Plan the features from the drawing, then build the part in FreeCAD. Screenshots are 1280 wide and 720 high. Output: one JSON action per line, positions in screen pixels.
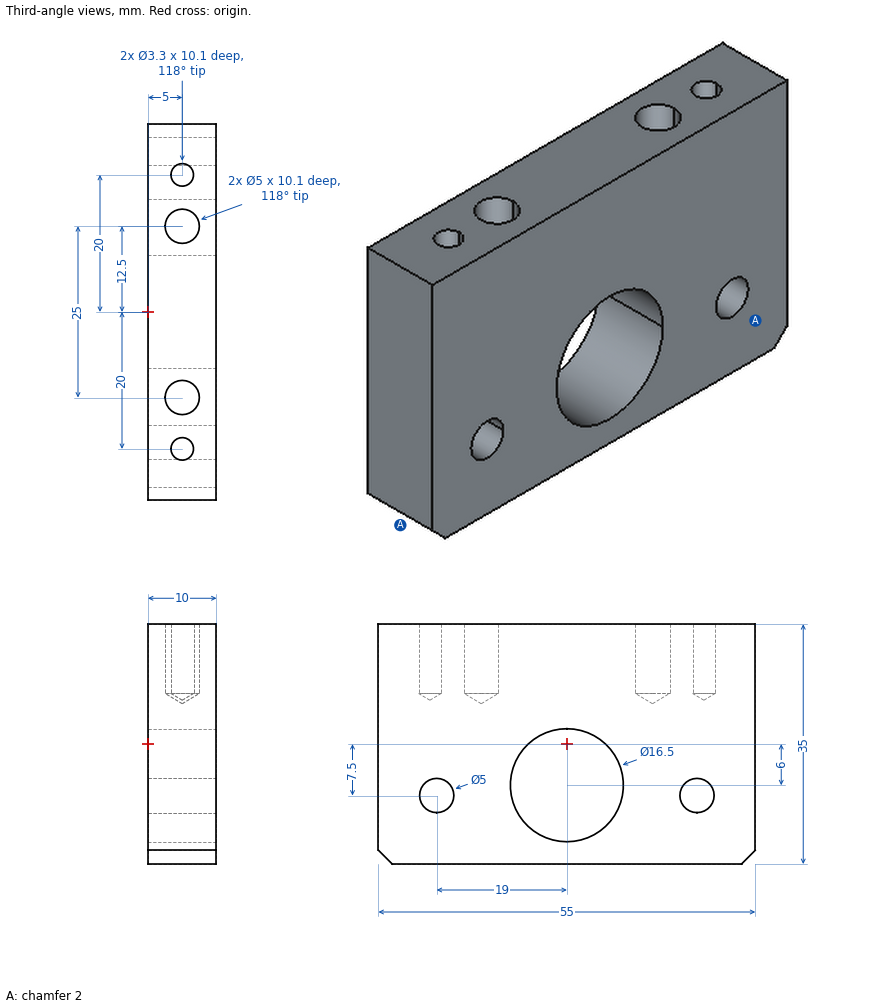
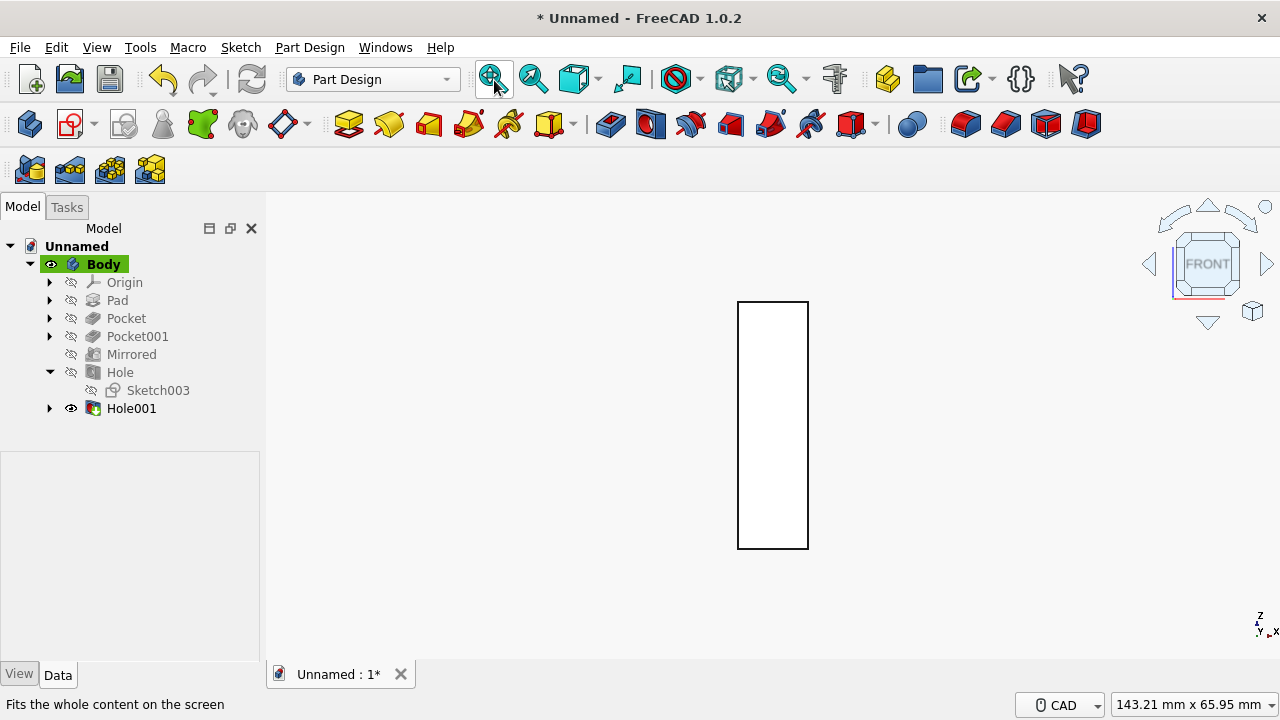
{"action": "left_click", "coordinate": [773, 548]}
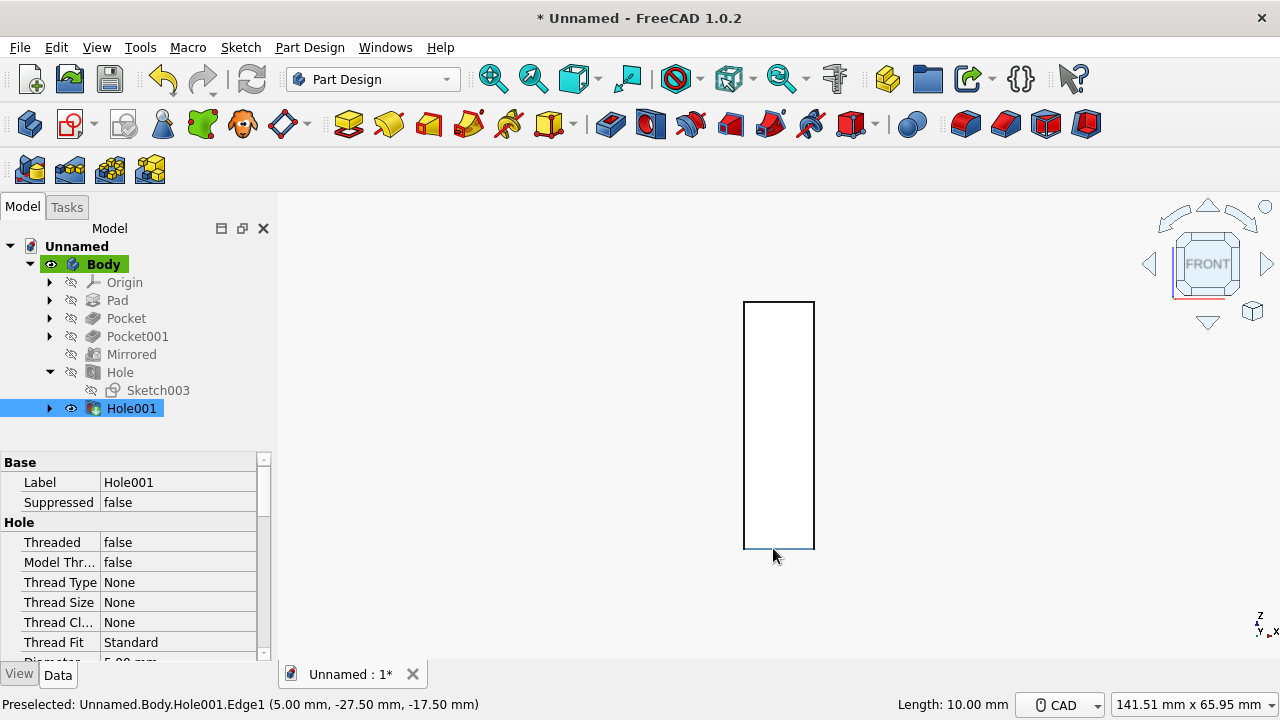
{"action": "key", "text": "3"}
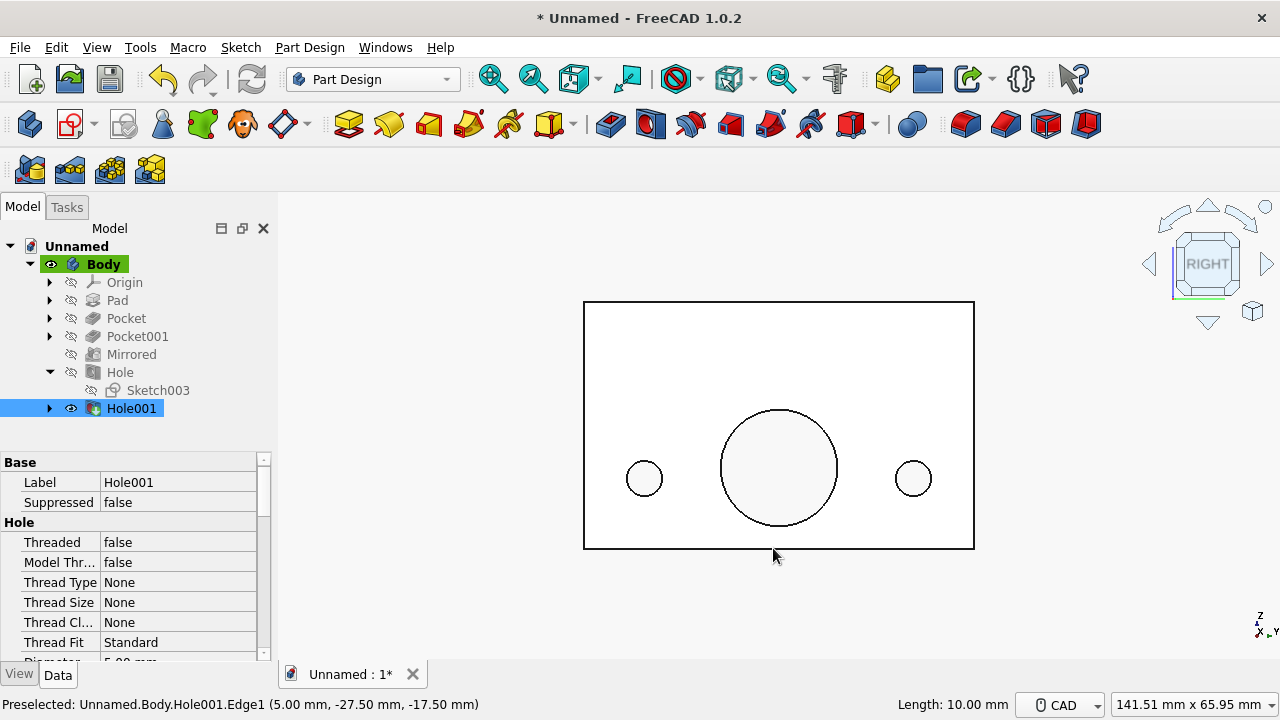
{"action": "key", "text": "5"}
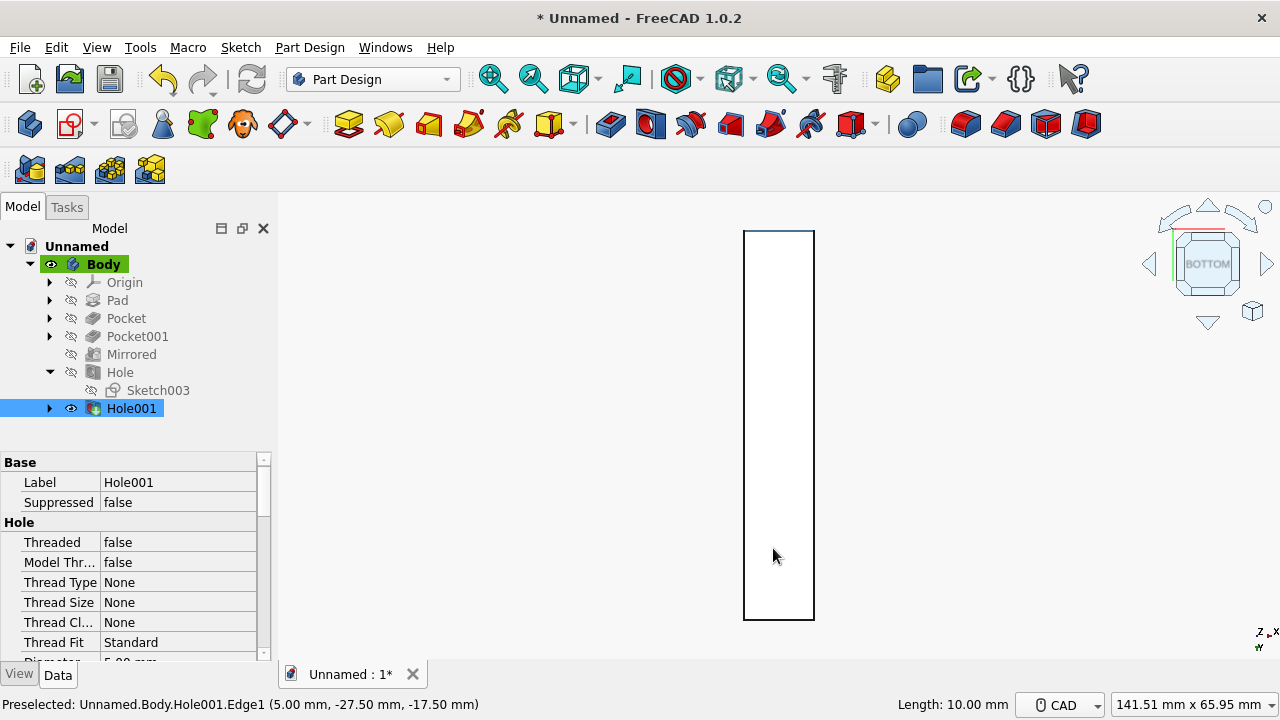
{"action": "left_click", "coordinate": [779, 619], "text": "ctrl"}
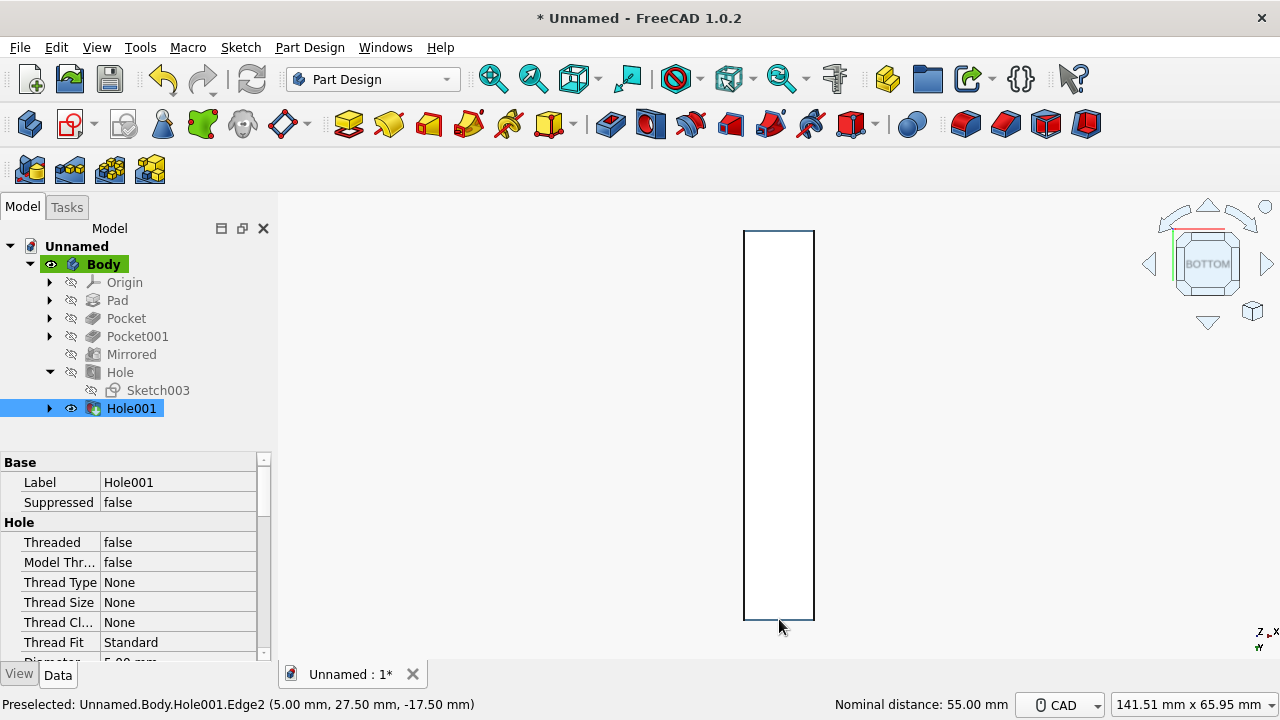
{"action": "left_click", "coordinate": [1006, 124]}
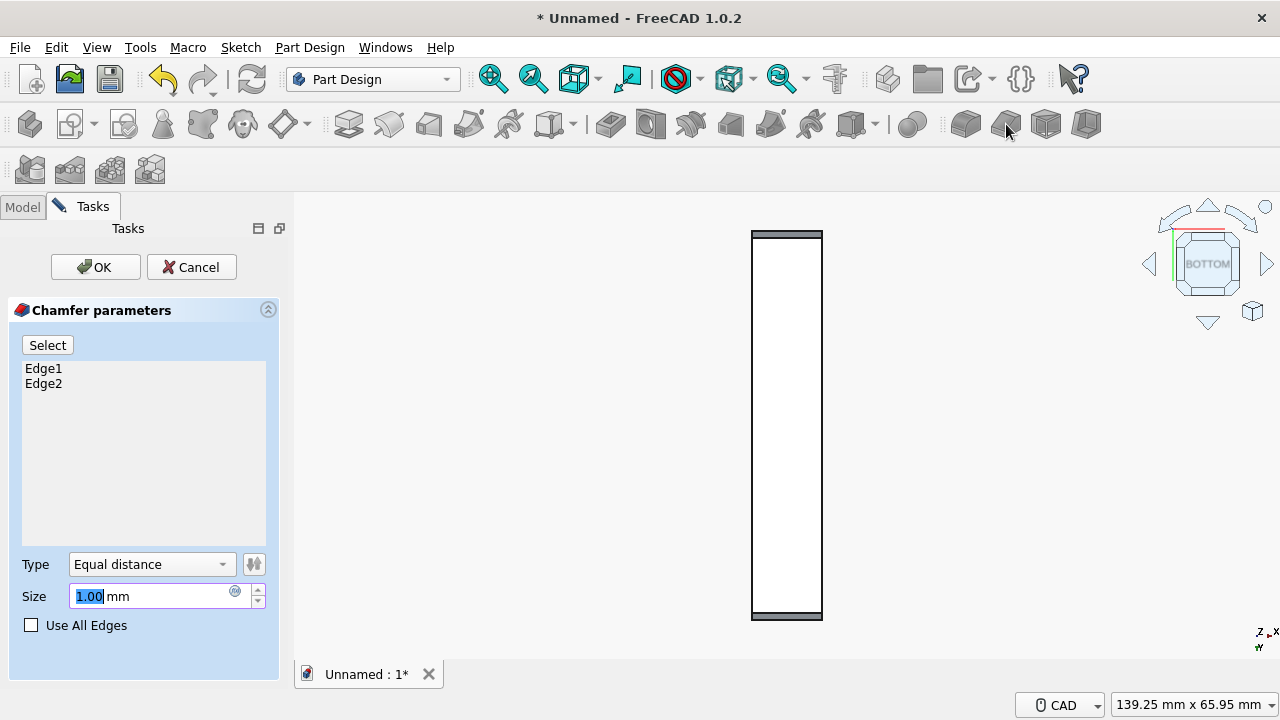
{"action": "type", "text": "2"}
{"action": "key", "text": "Tab"}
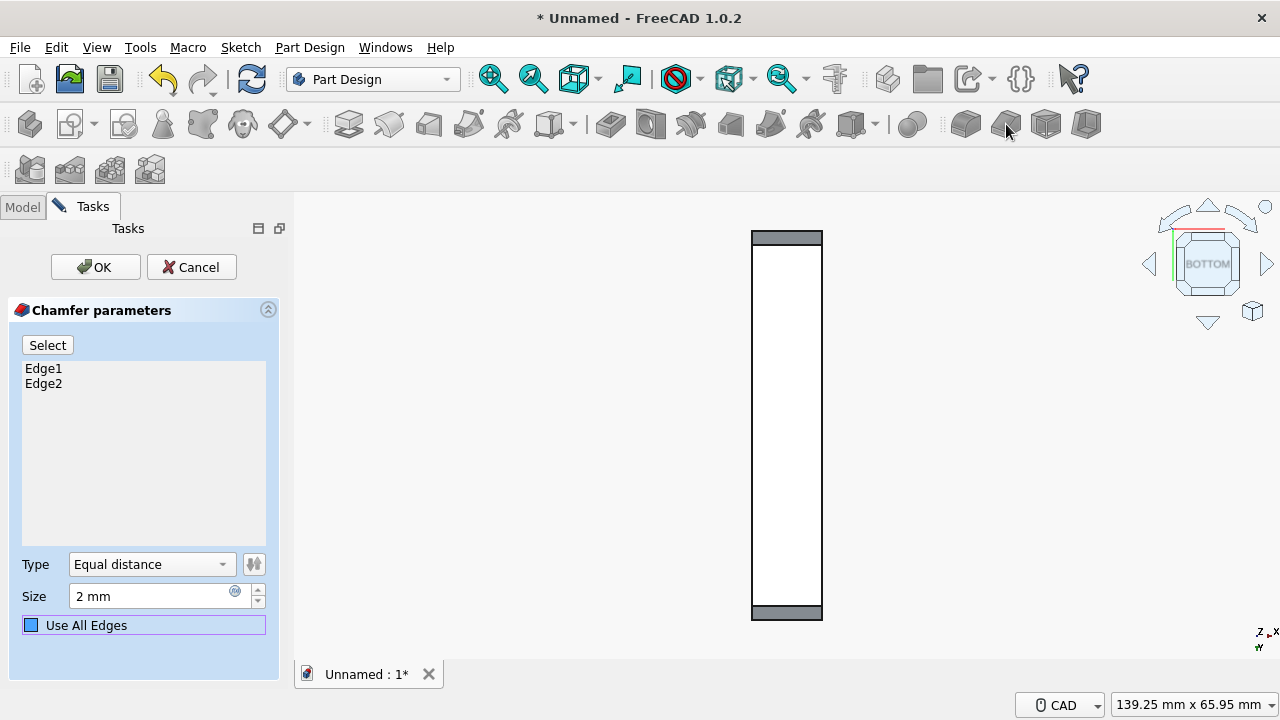
{"action": "left_click", "coordinate": [96, 267]}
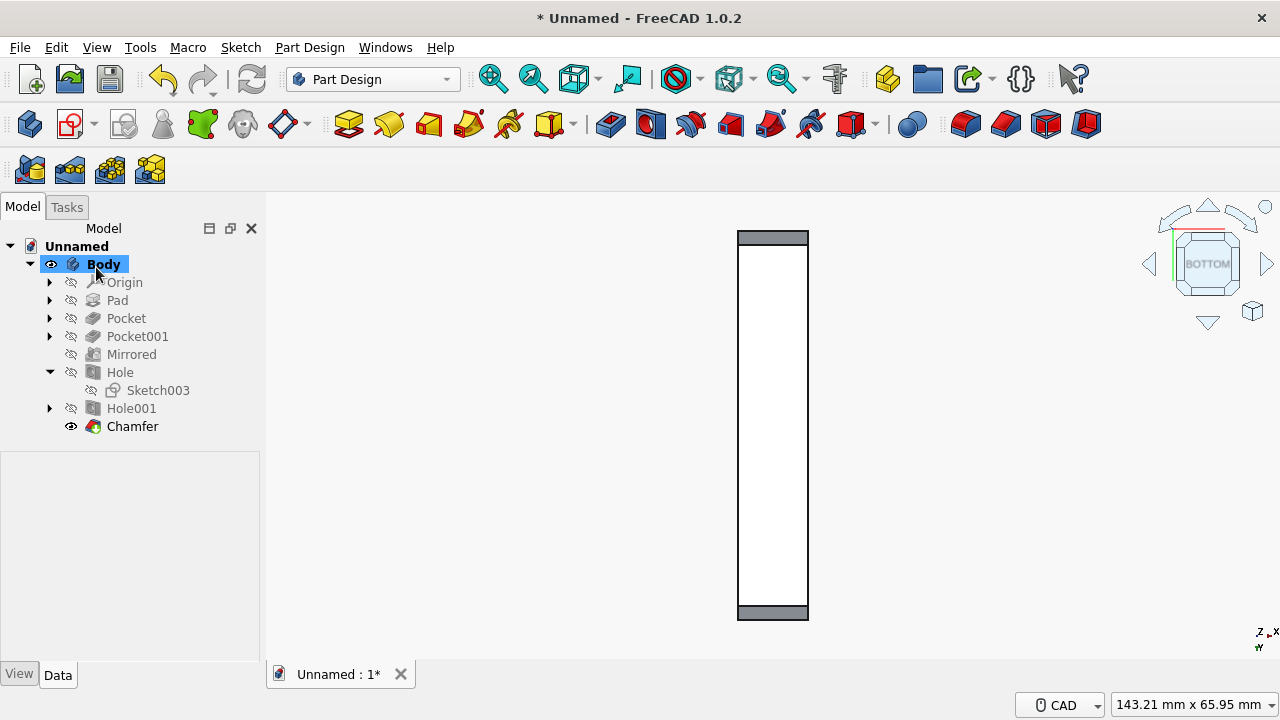
{"action": "key", "text": "0"}